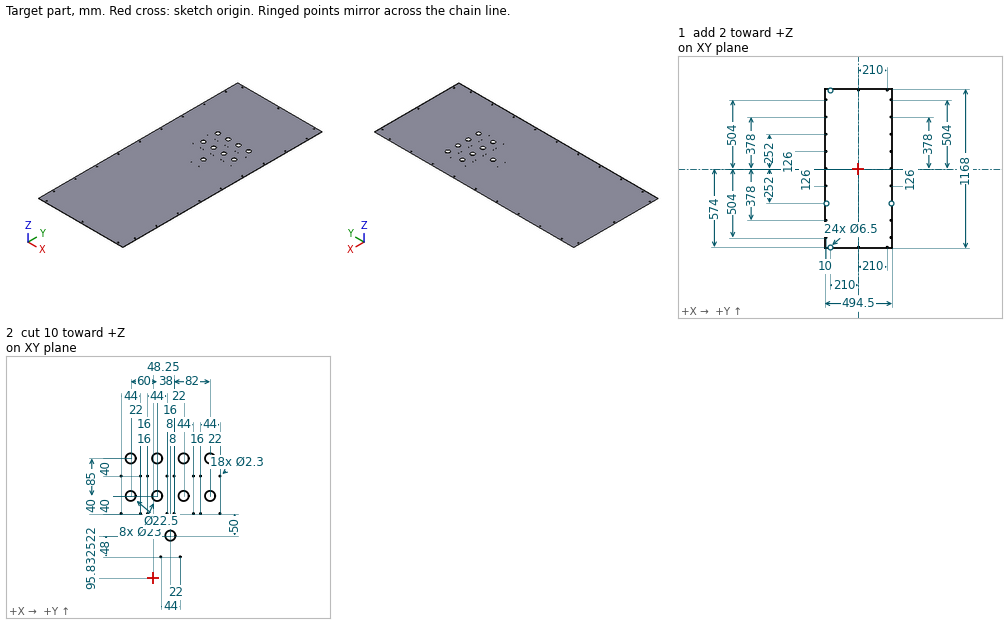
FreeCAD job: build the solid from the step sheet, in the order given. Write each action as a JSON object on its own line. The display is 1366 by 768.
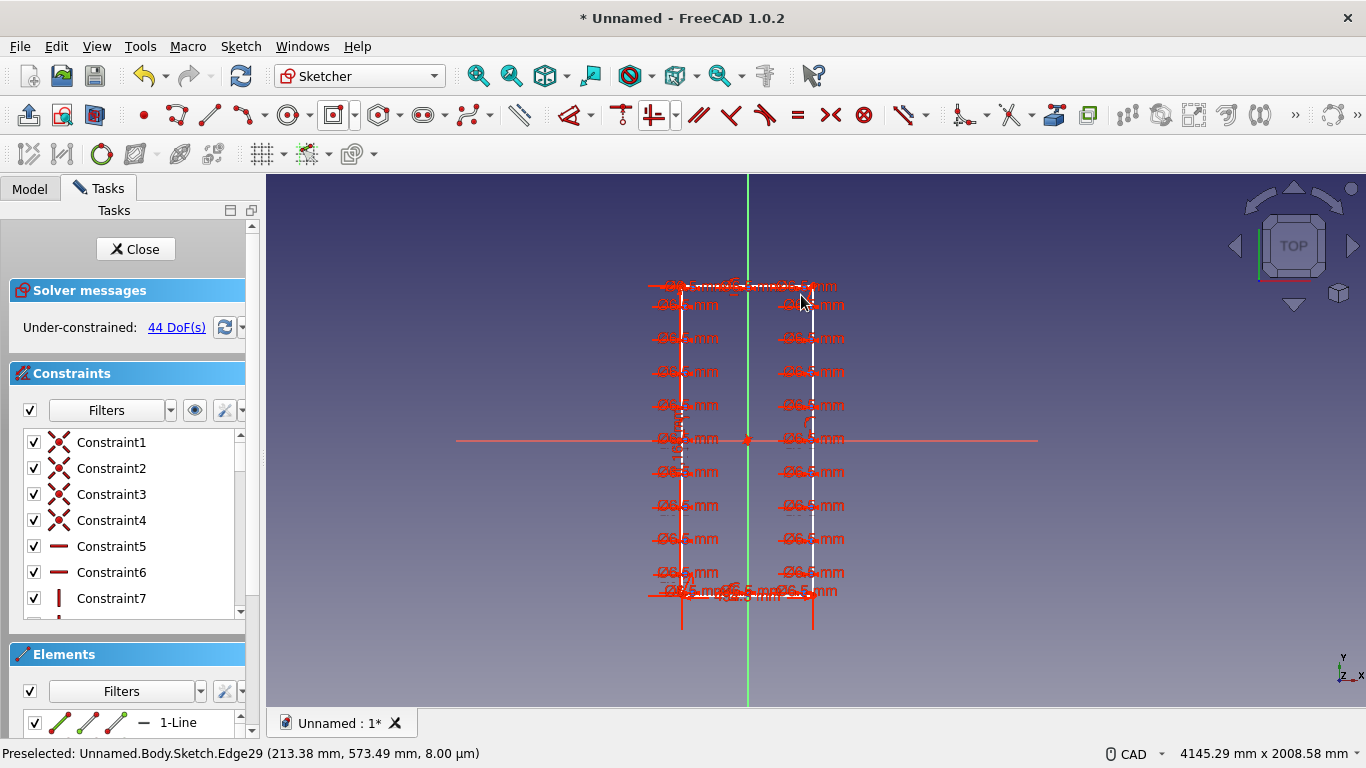
{"action": "left_click", "coordinate": [685, 575]}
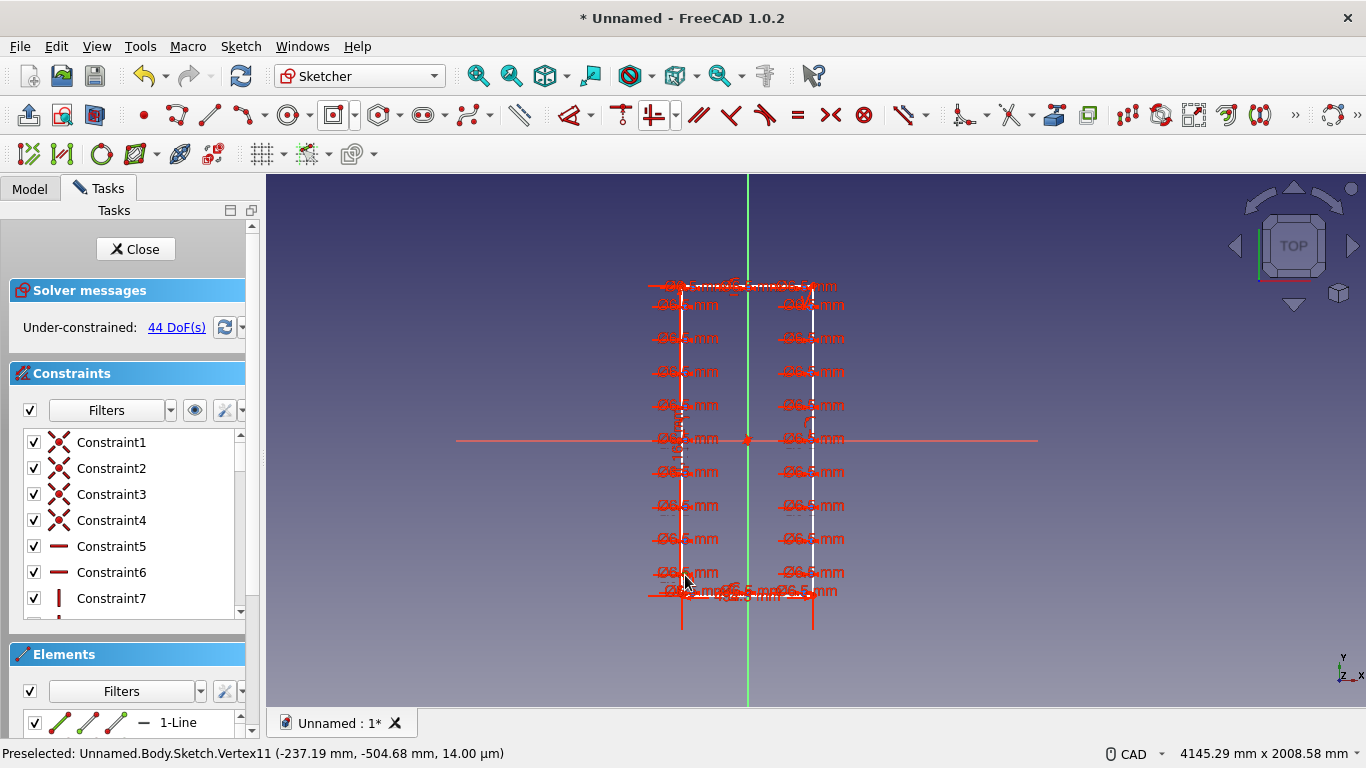
{"action": "left_click", "coordinate": [685, 541]}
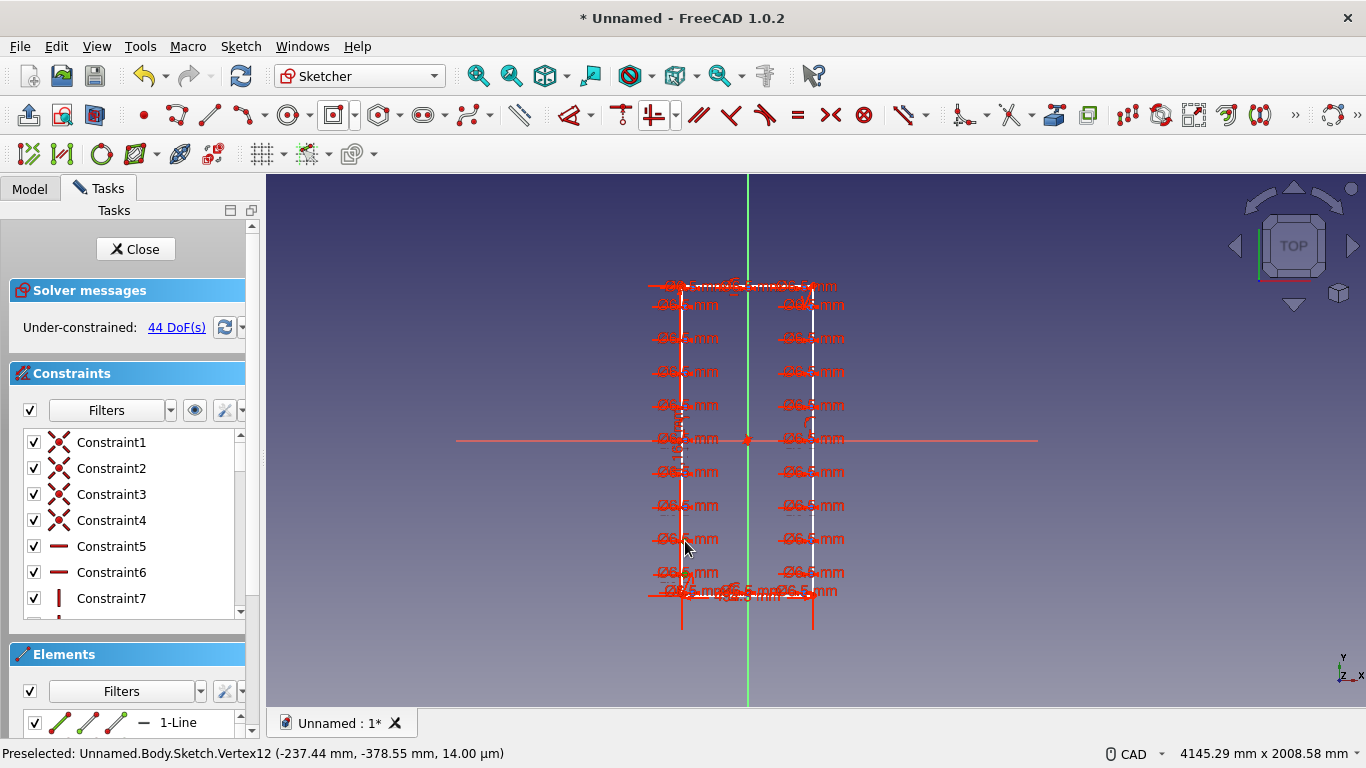
{"action": "left_click", "coordinate": [676, 116]}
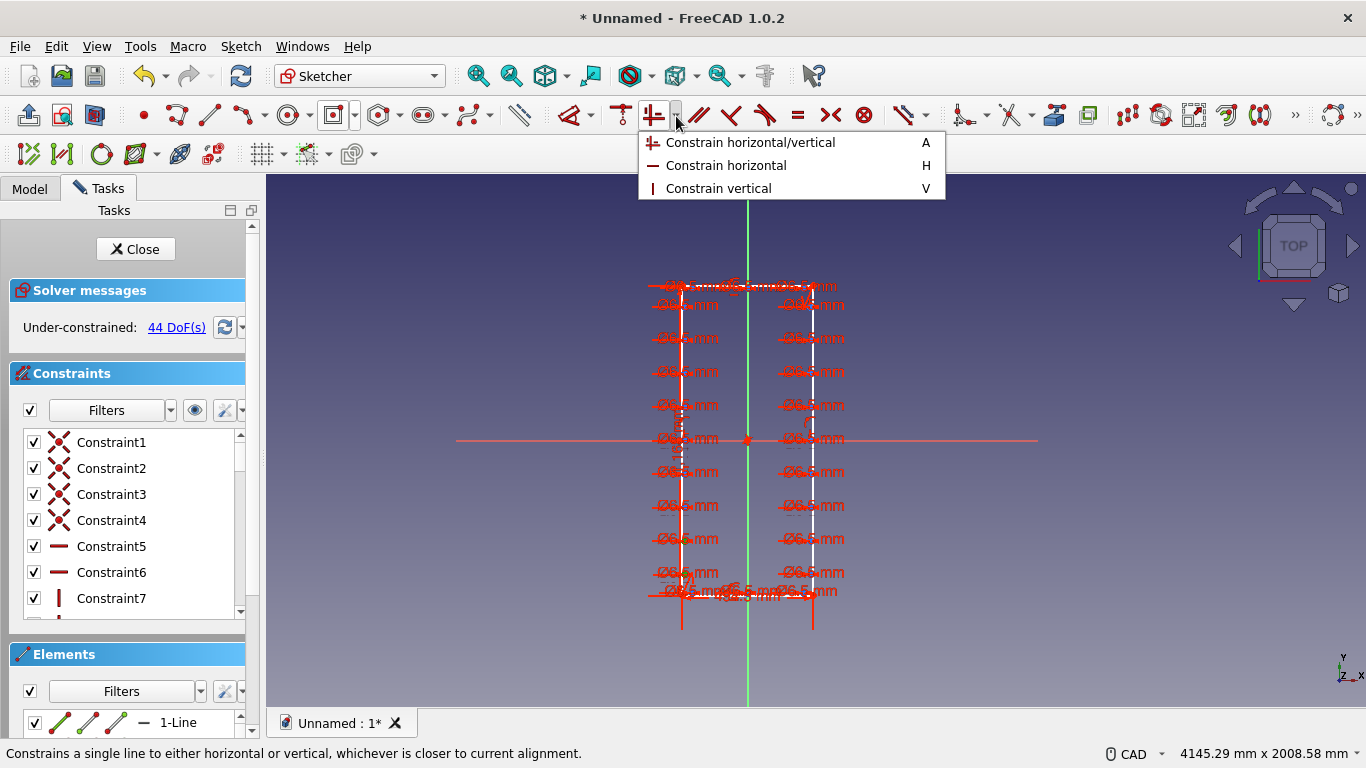
{"action": "left_click", "coordinate": [792, 188]}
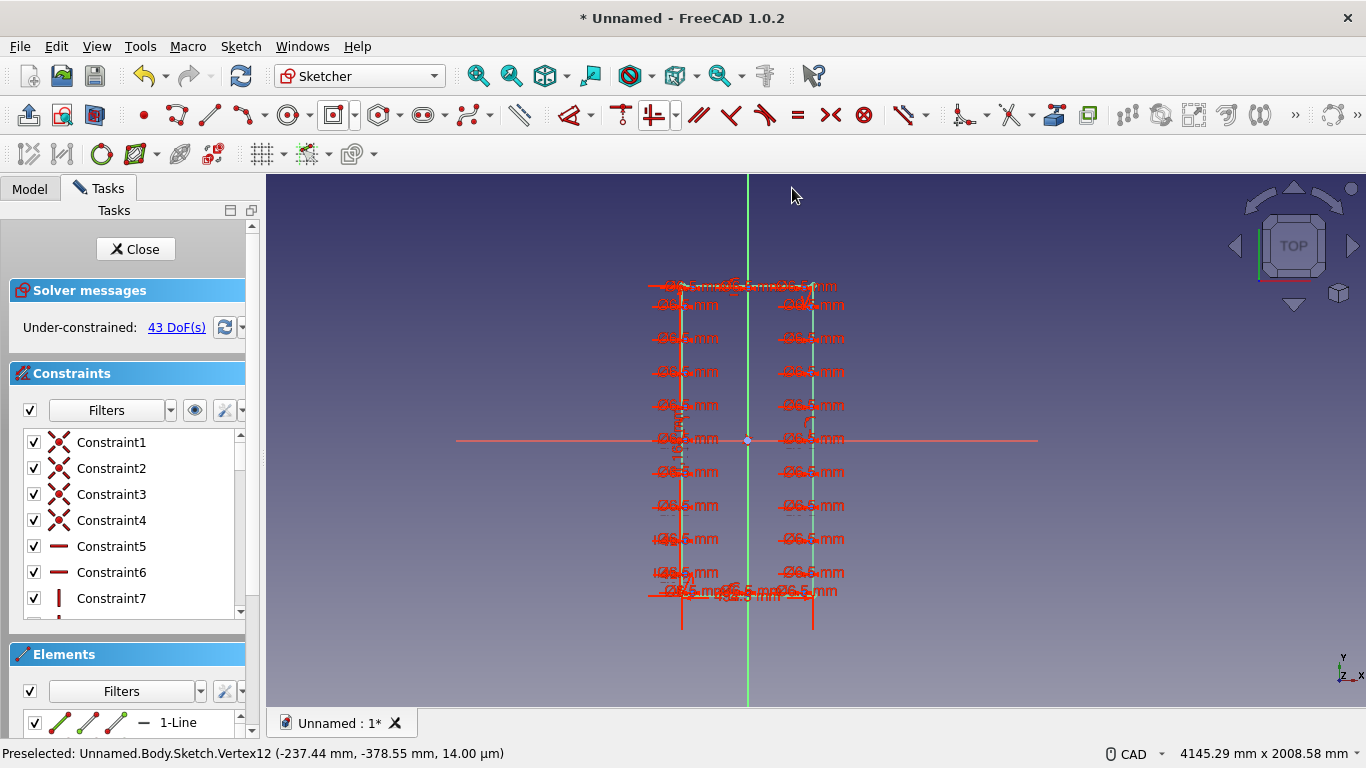
{"action": "left_click", "coordinate": [685, 541]}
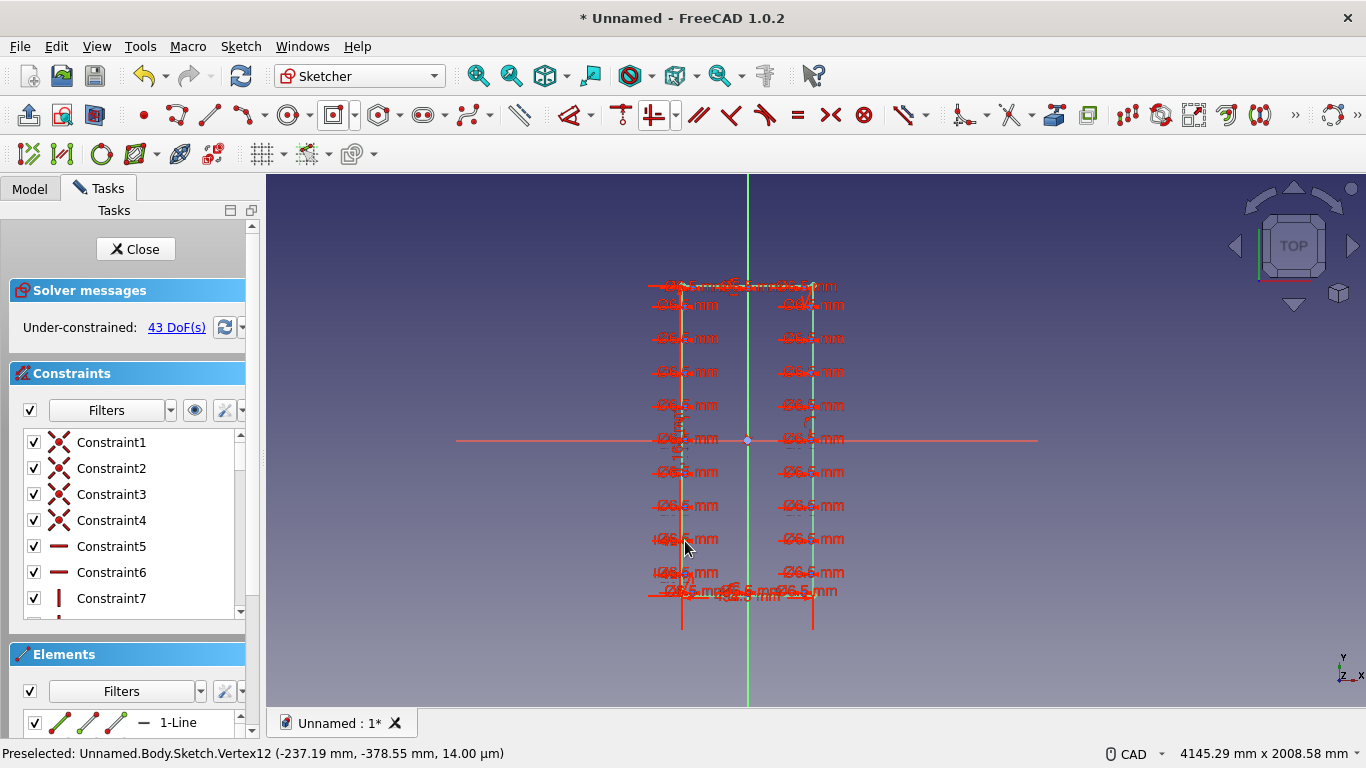
{"action": "left_click", "coordinate": [685, 508]}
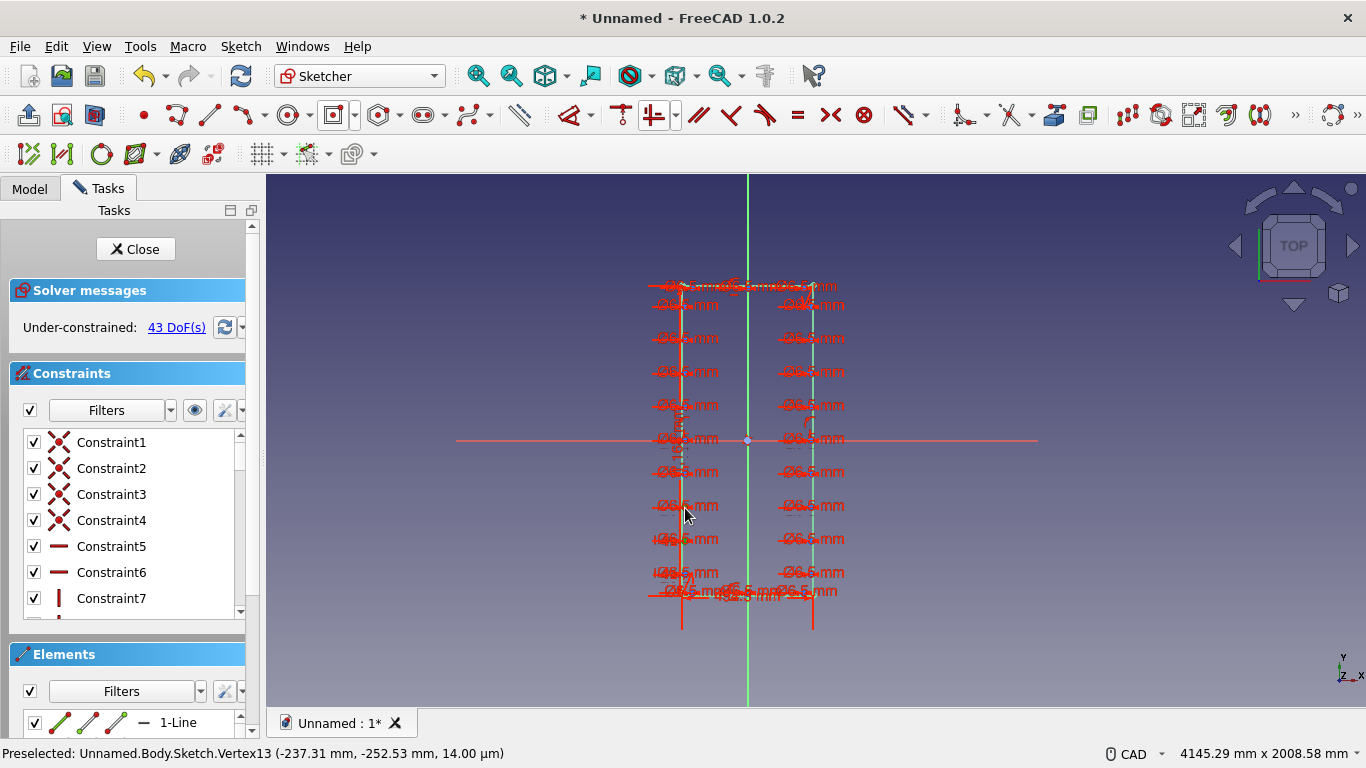
{"action": "left_click", "coordinate": [676, 116]}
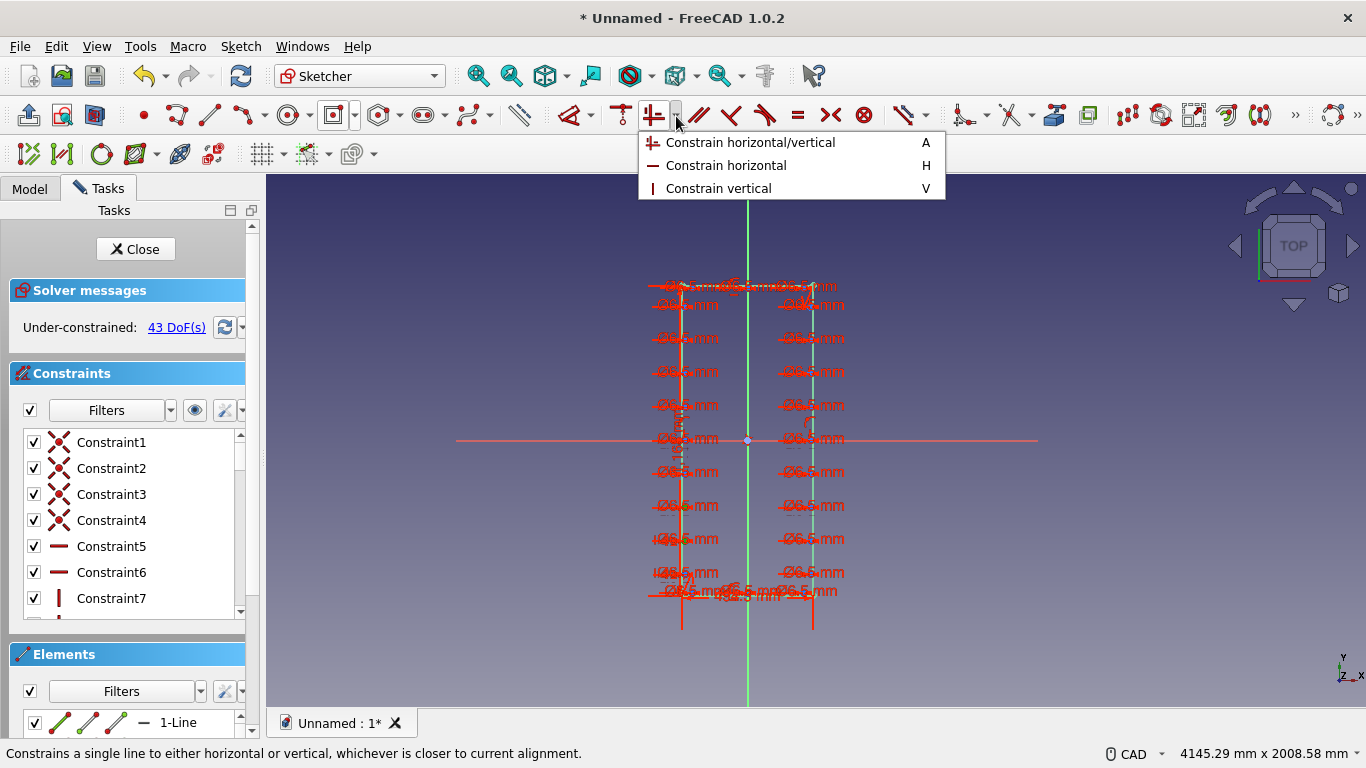
{"action": "left_click", "coordinate": [792, 188]}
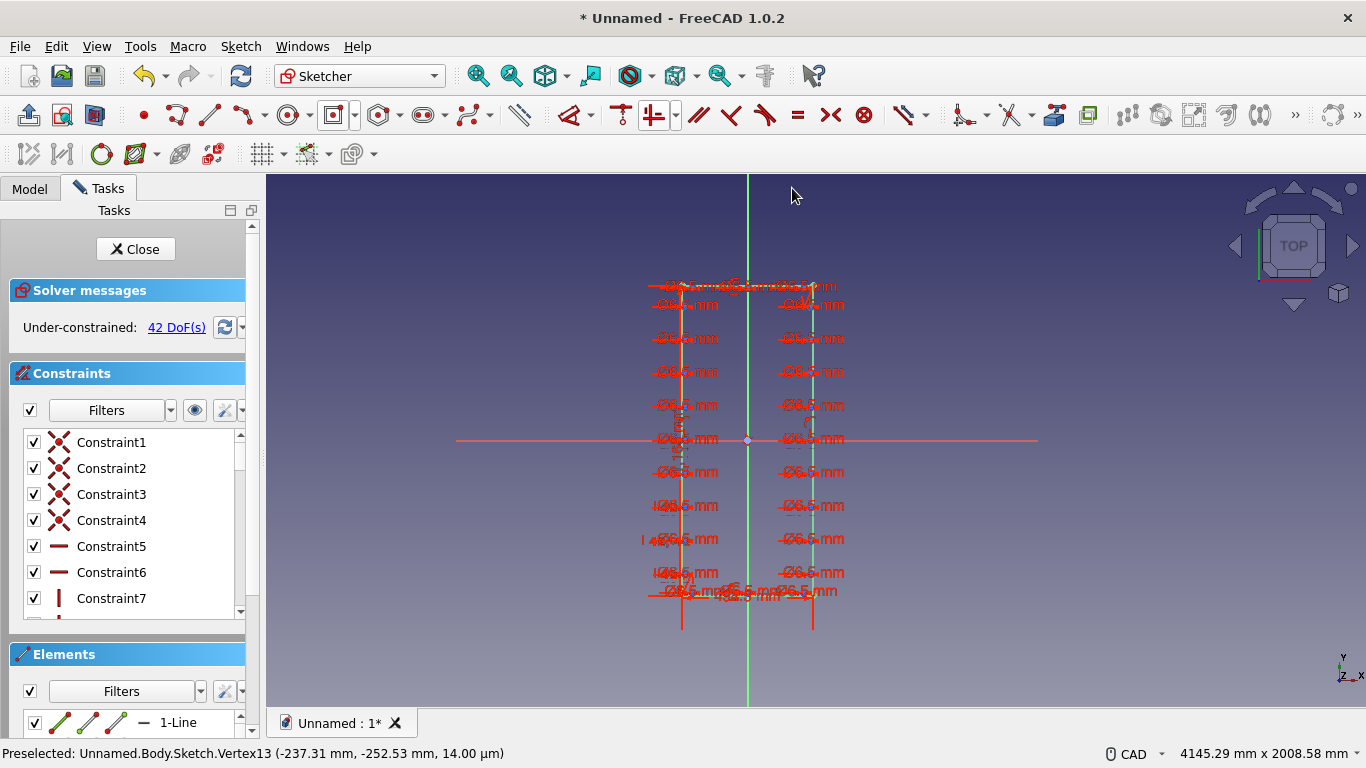
{"action": "left_click", "coordinate": [685, 508]}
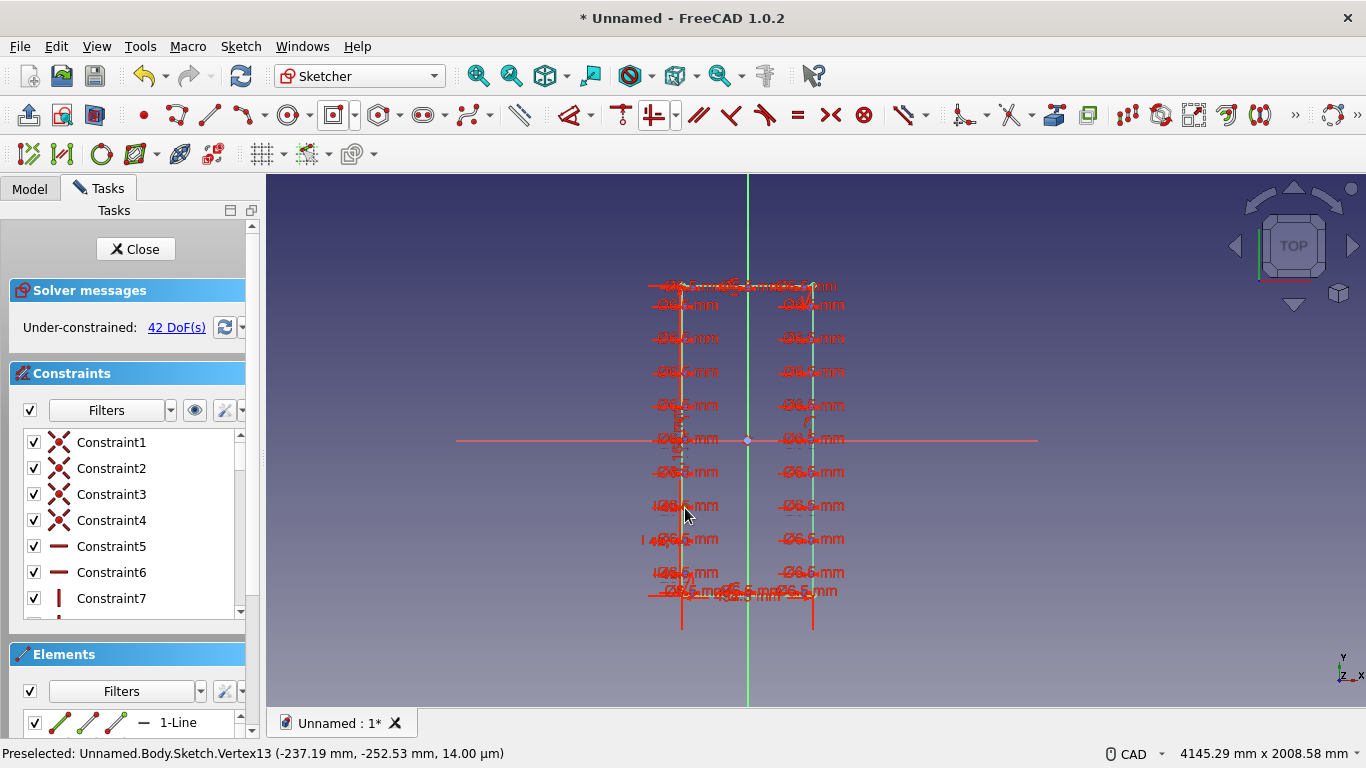
{"action": "left_click", "coordinate": [685, 474]}